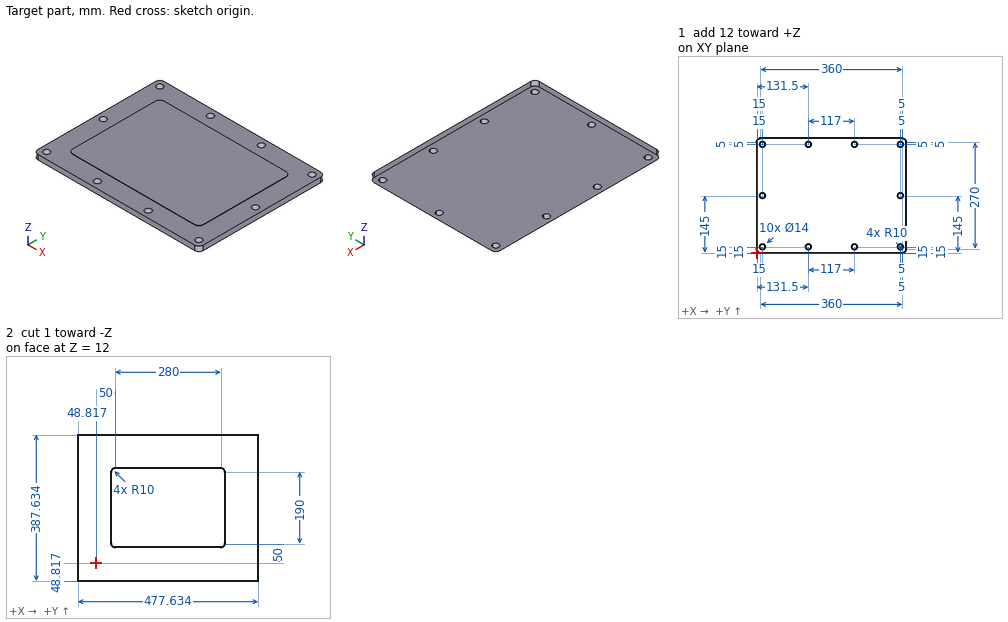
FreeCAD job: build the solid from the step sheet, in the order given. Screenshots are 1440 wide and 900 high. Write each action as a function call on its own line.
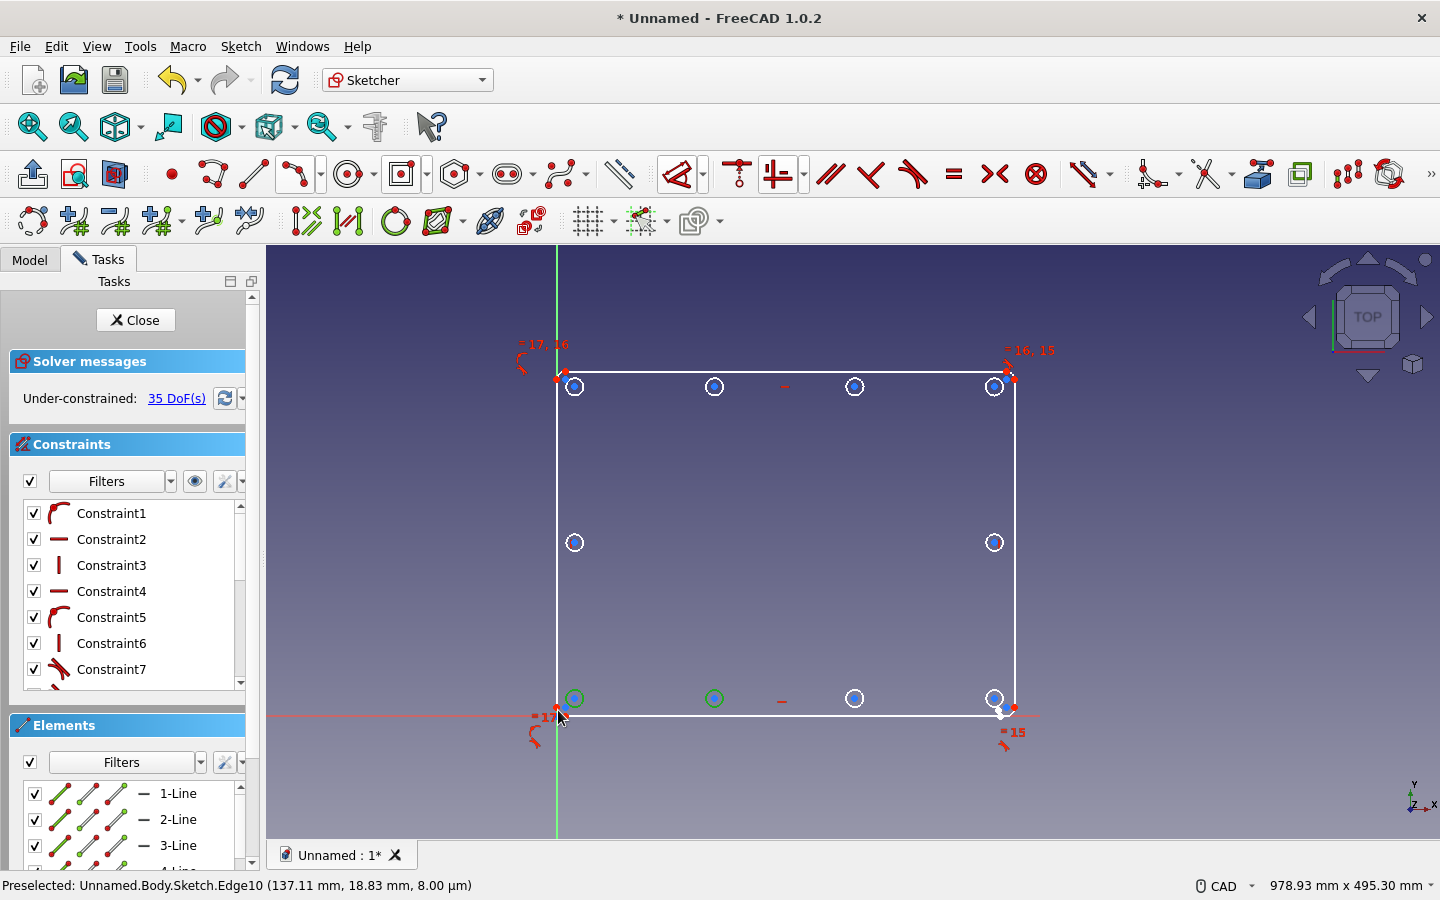
scroll(861, 692, up, 3)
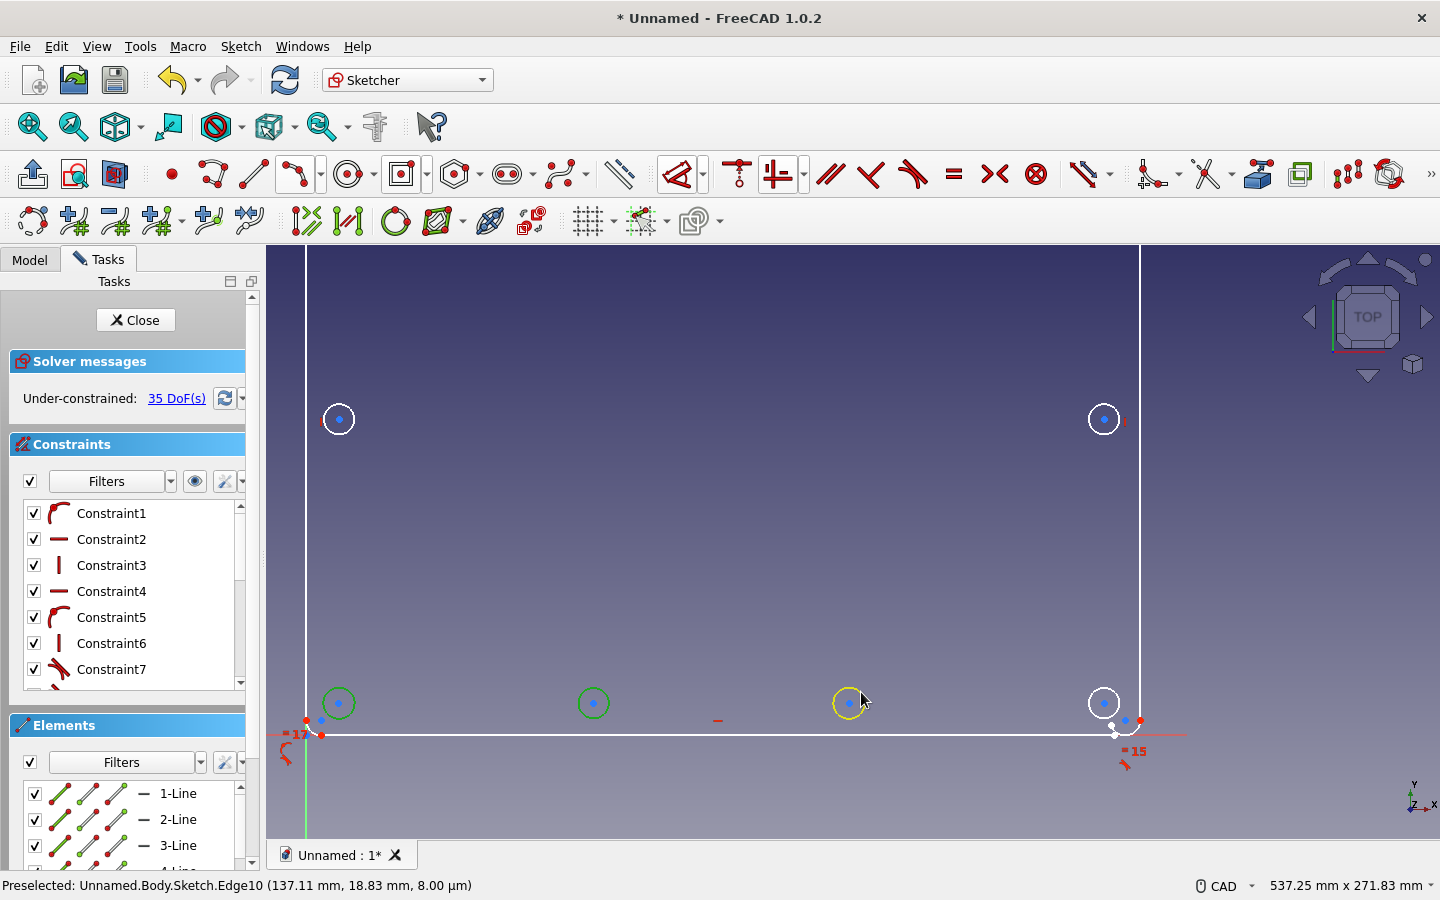
click(860, 692)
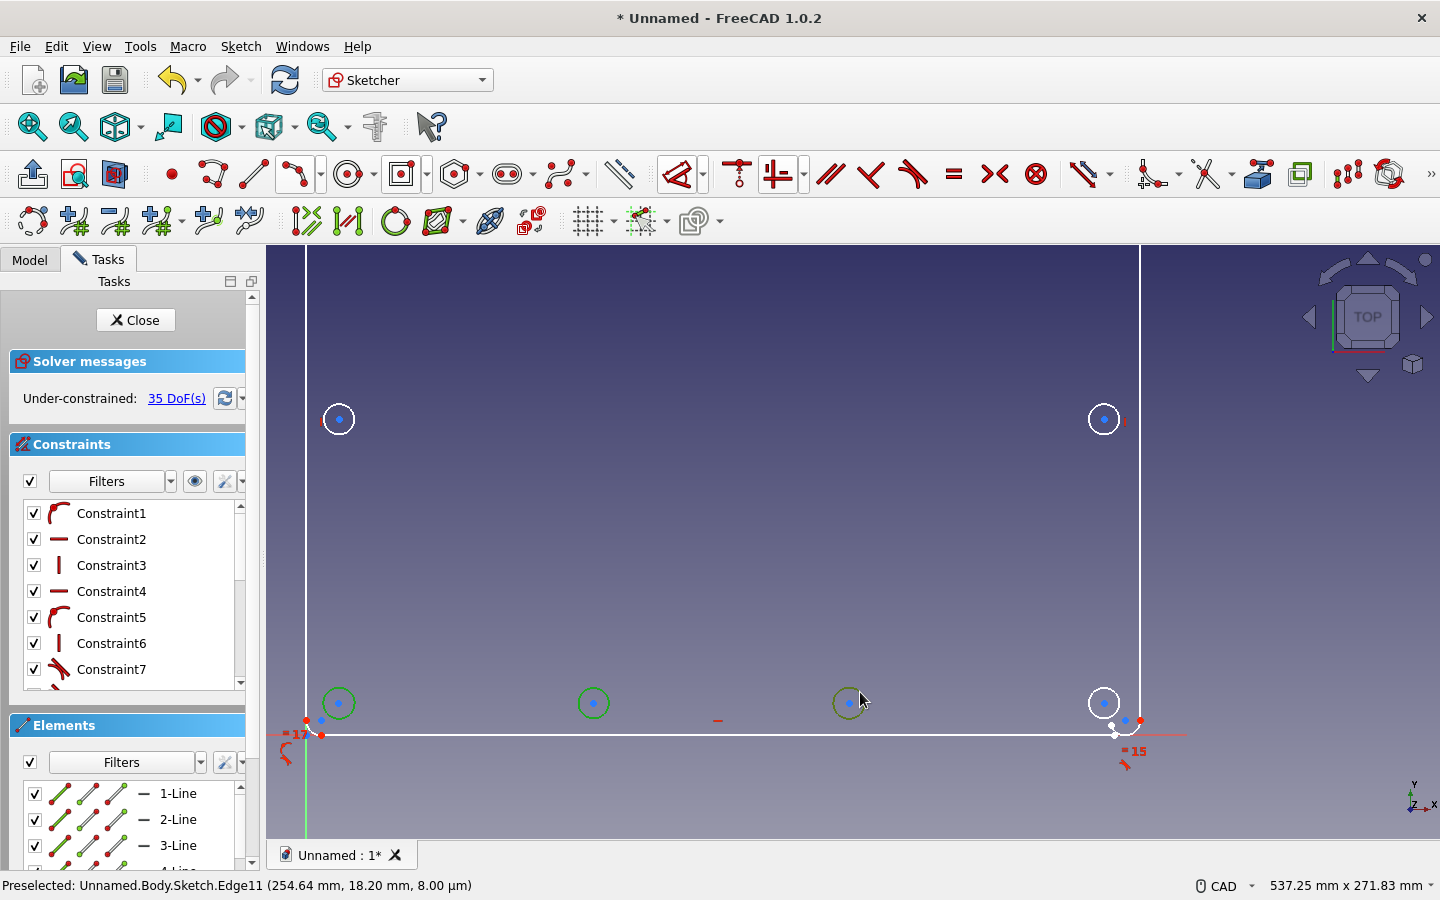
click(1115, 692)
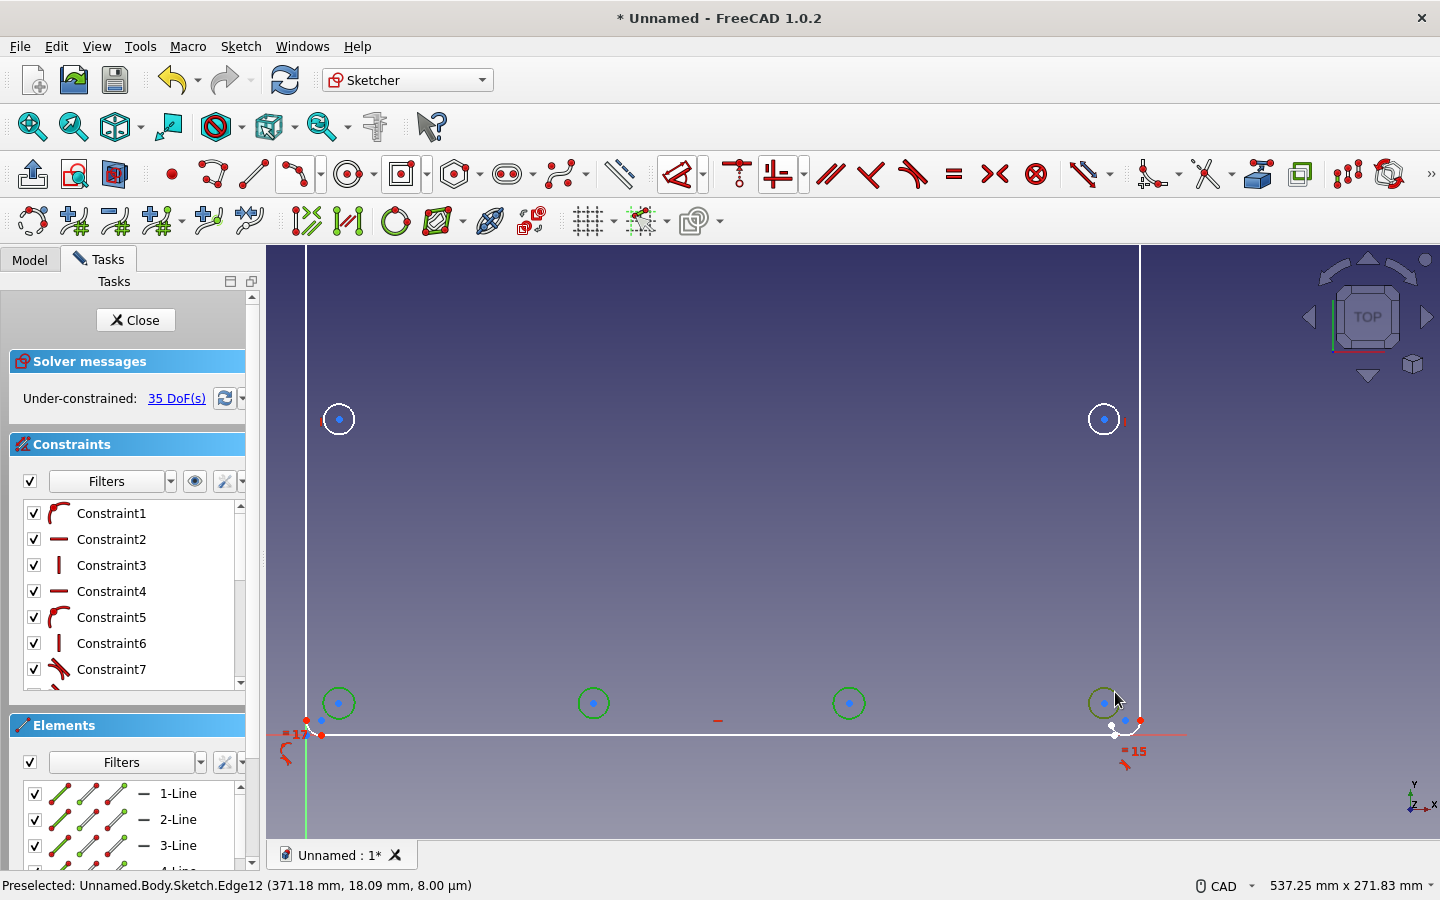
click(350, 409)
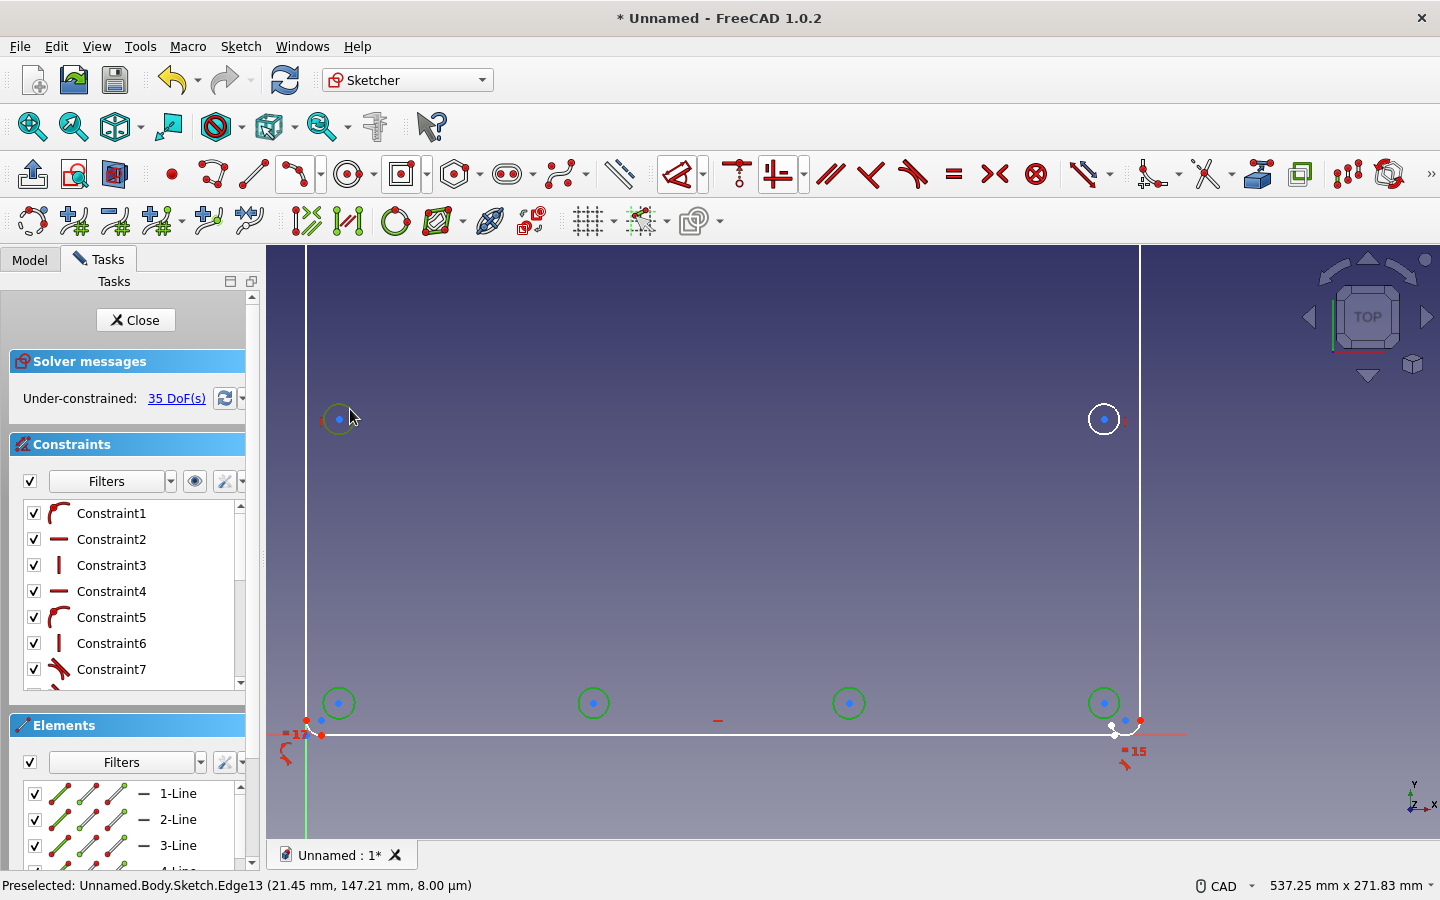
scroll(861, 692, down, 3)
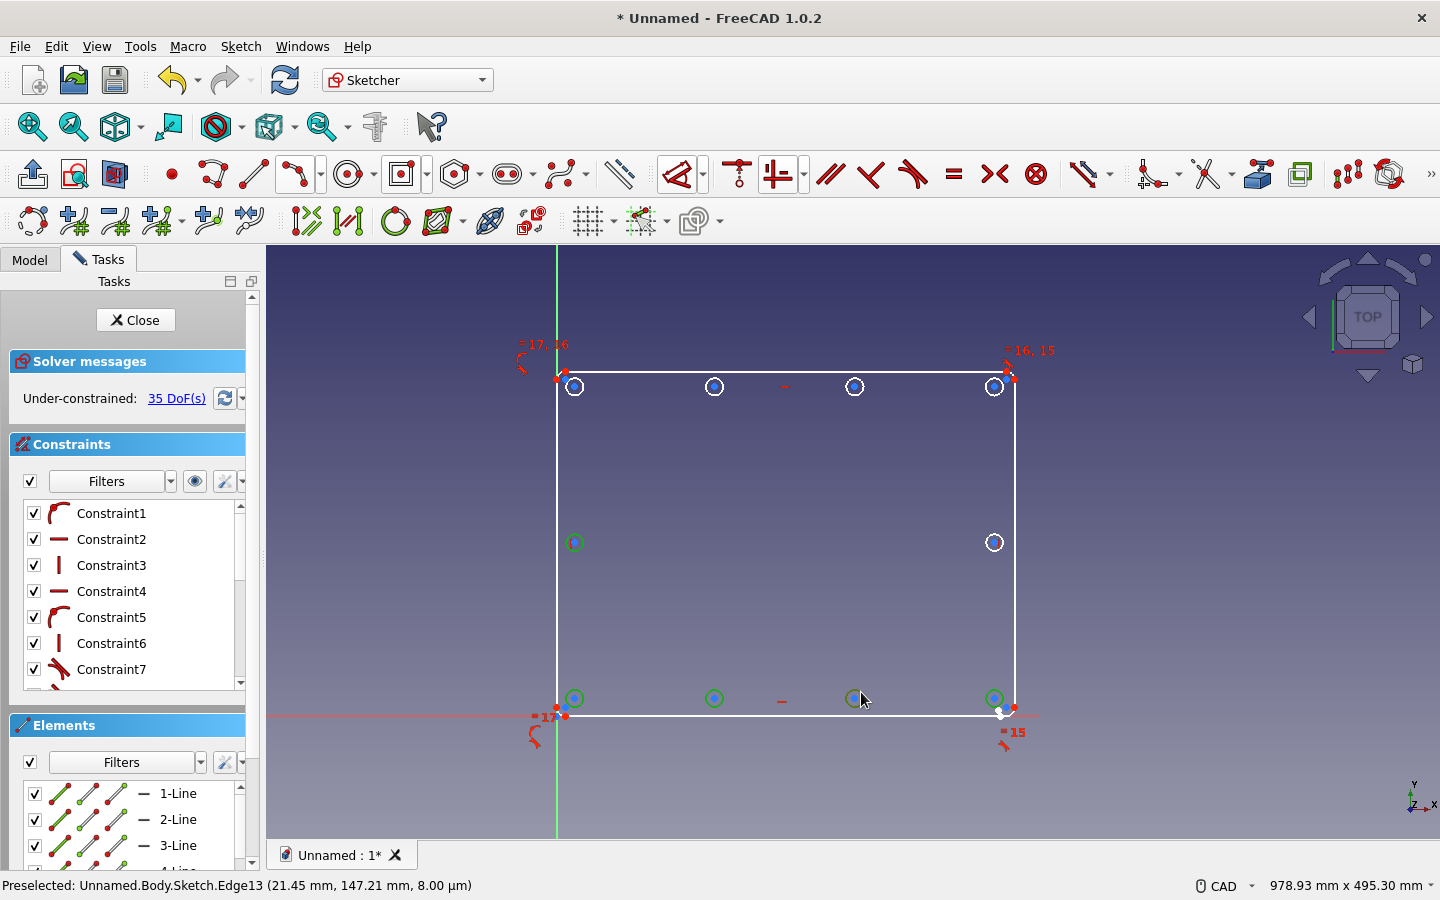
scroll(581, 381, up, 3)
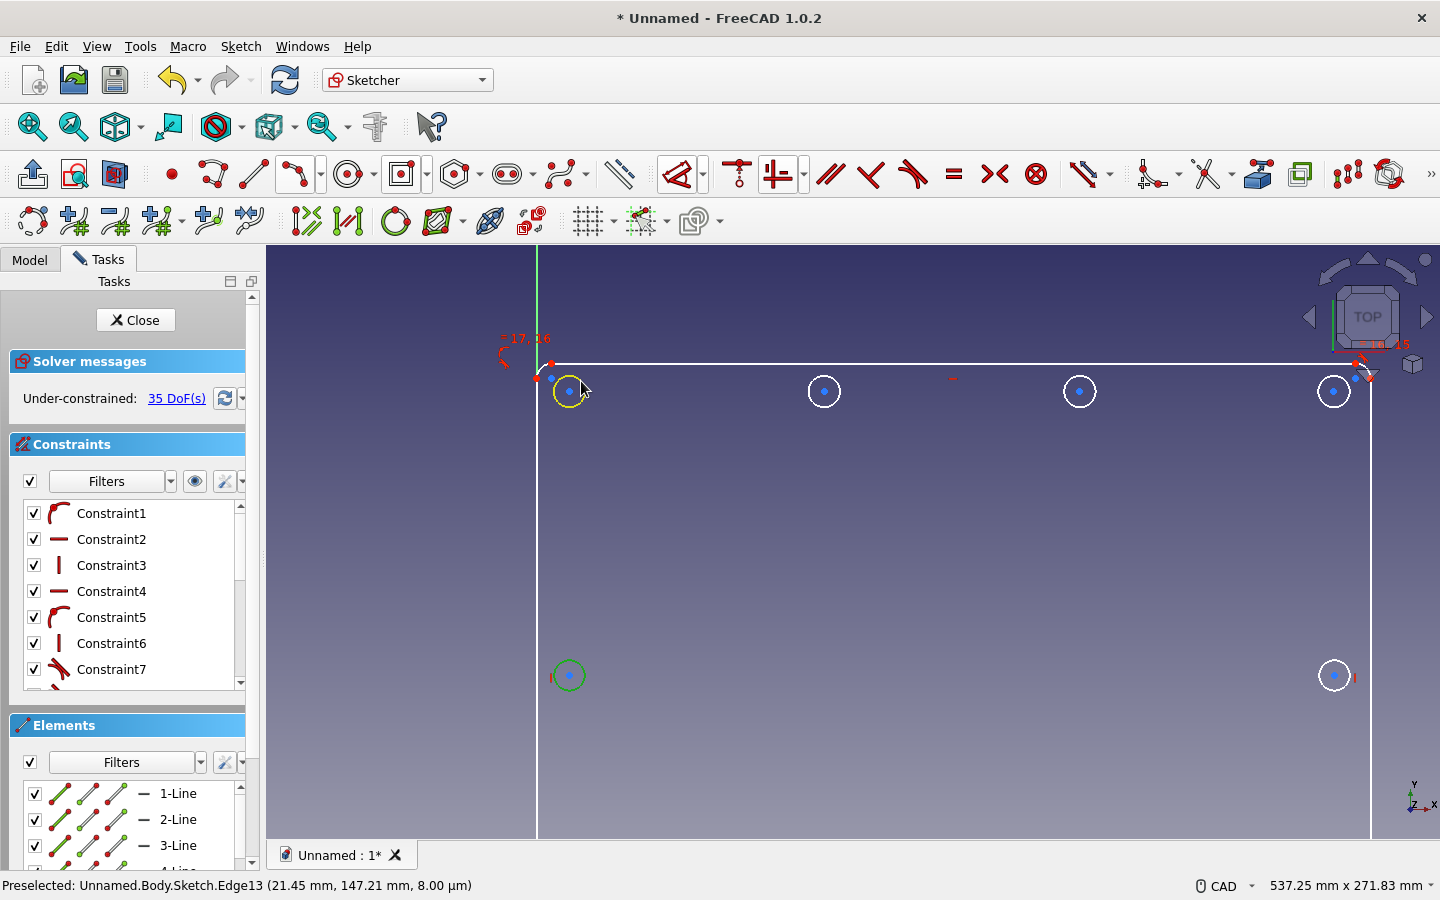
click(581, 380)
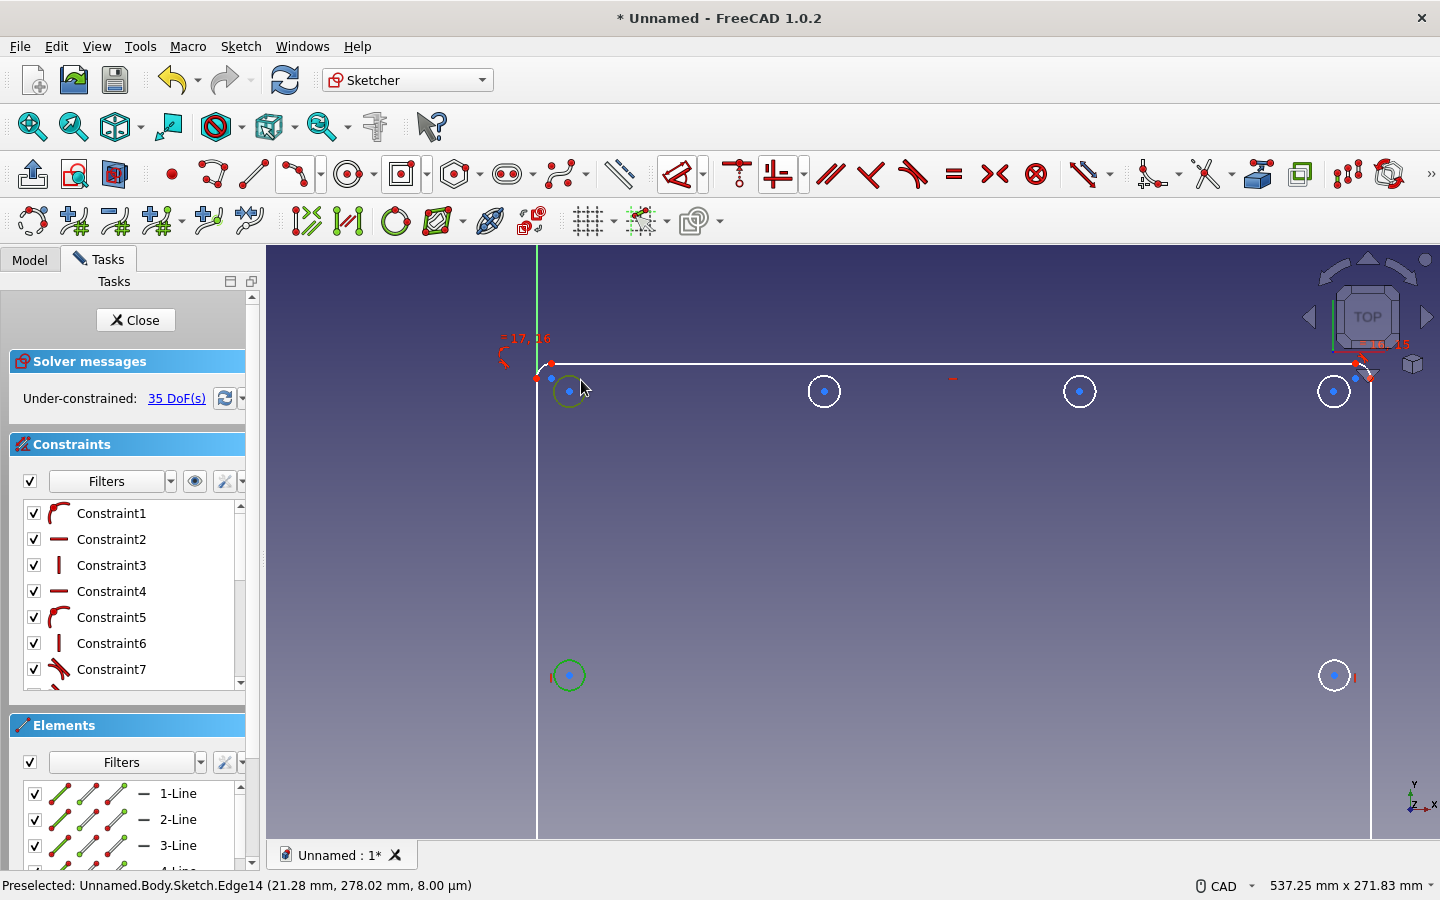
click(835, 380)